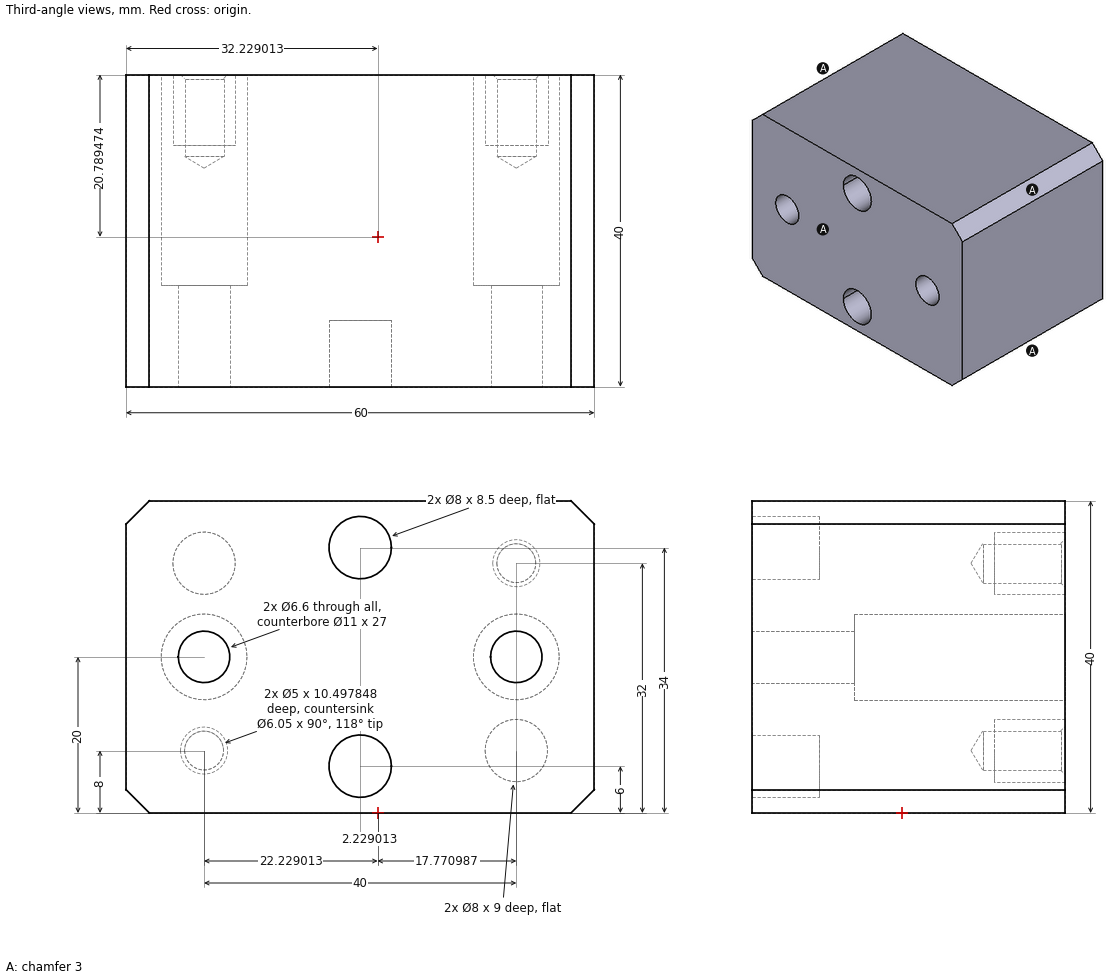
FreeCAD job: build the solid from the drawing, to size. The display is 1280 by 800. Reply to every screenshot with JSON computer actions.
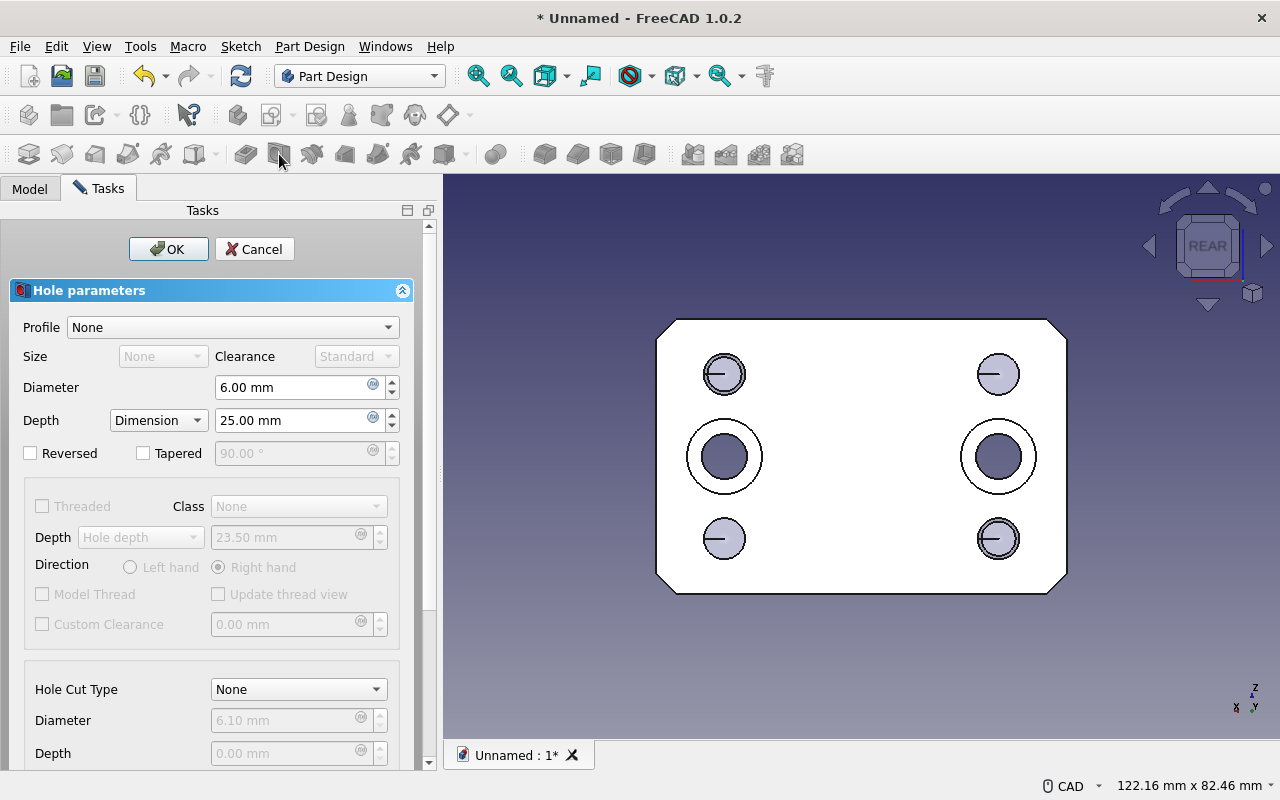
{"action": "triple_click", "coordinate": [300, 388]}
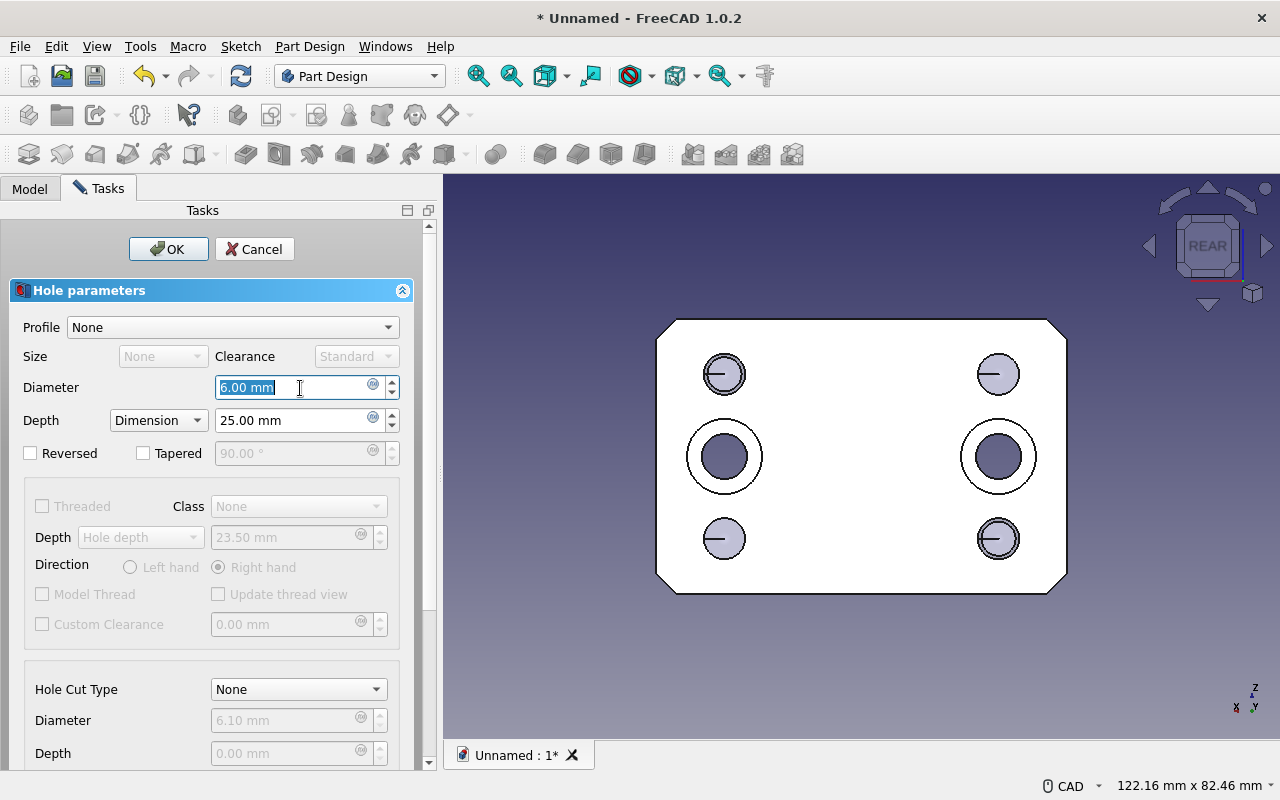
{"action": "type", "text": "8"}
{"action": "key", "text": "Tab"}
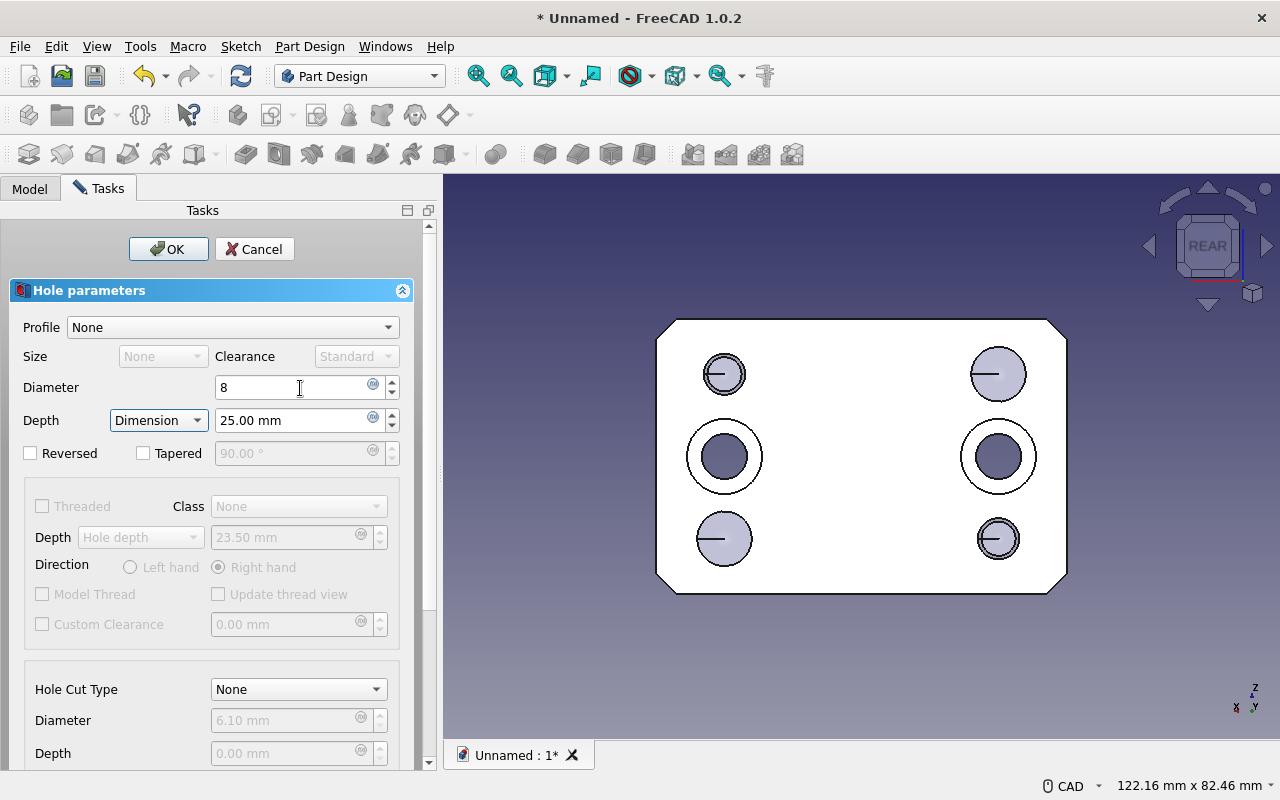
{"action": "triple_click", "coordinate": [300, 420]}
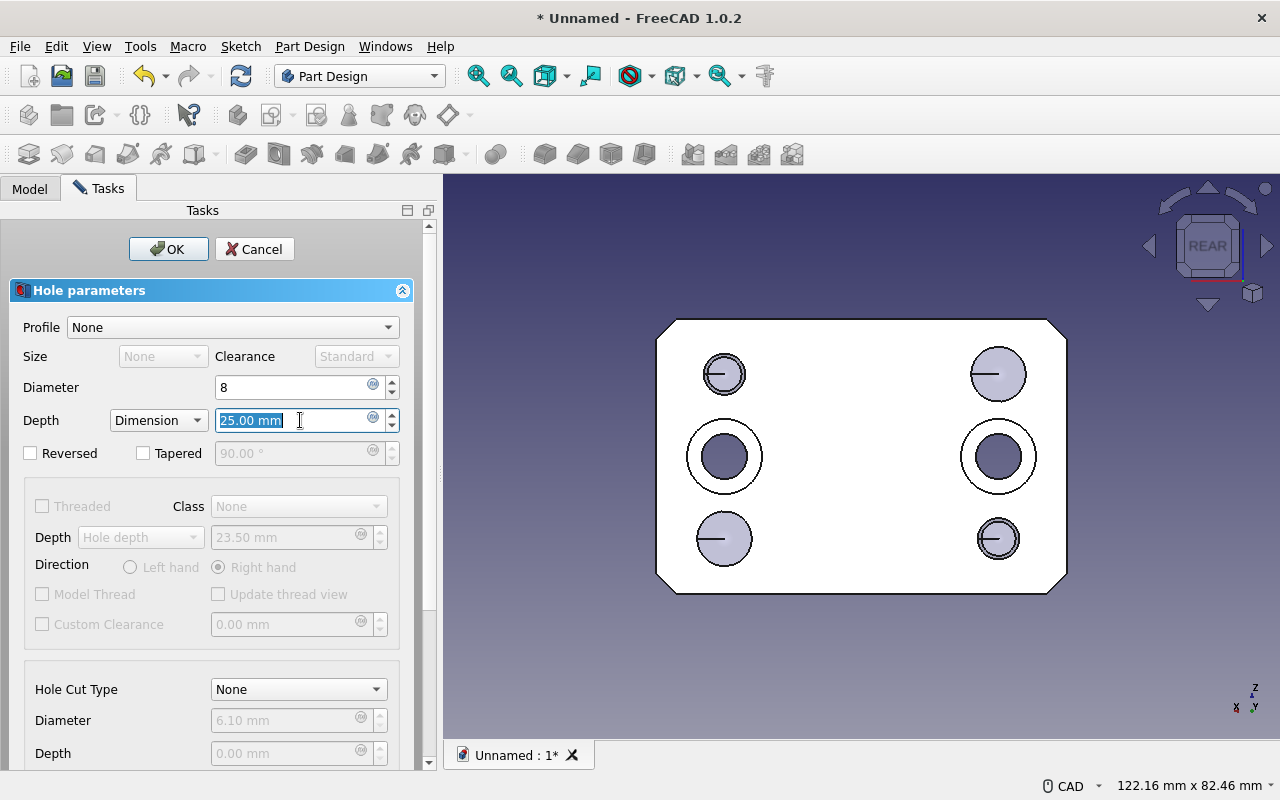
{"action": "type", "text": "9"}
{"action": "key", "text": "Tab"}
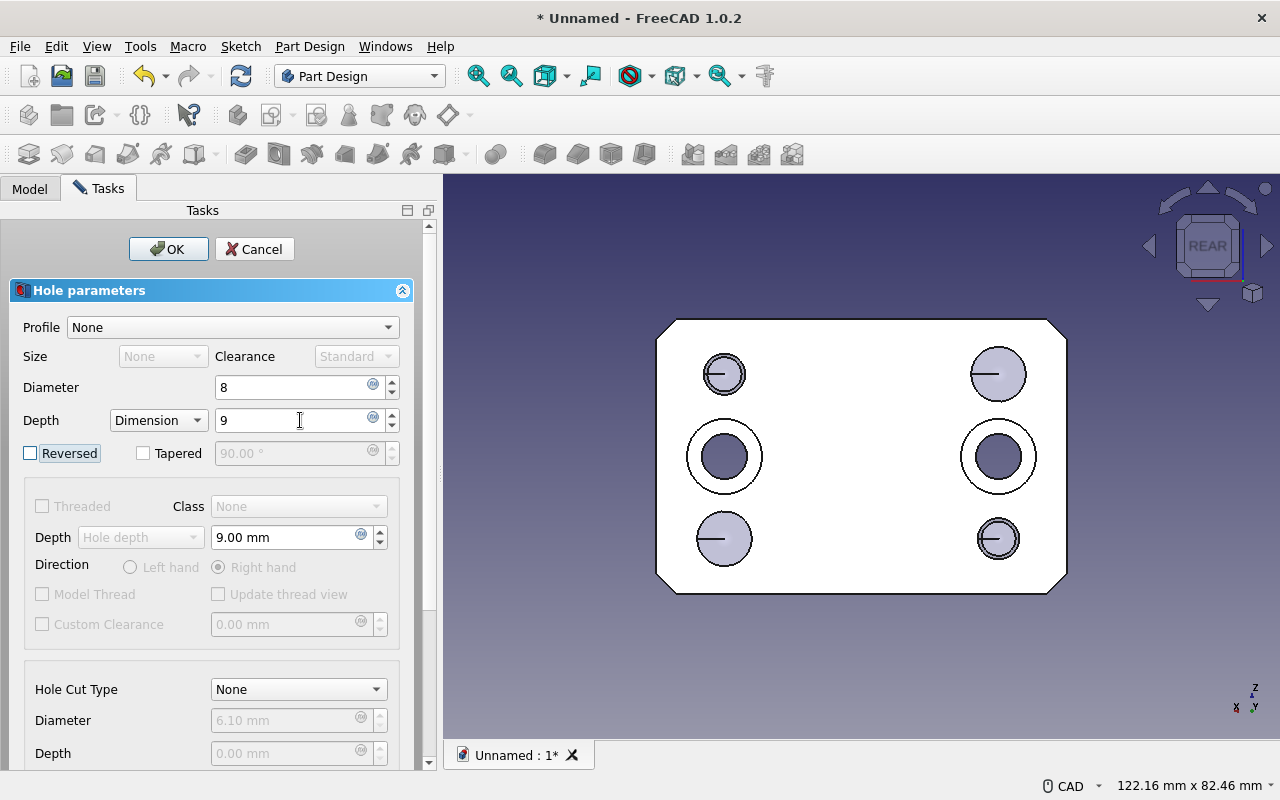
{"action": "scroll", "coordinate": [429, 495], "scroll_direction": "down", "scroll_amount": 3}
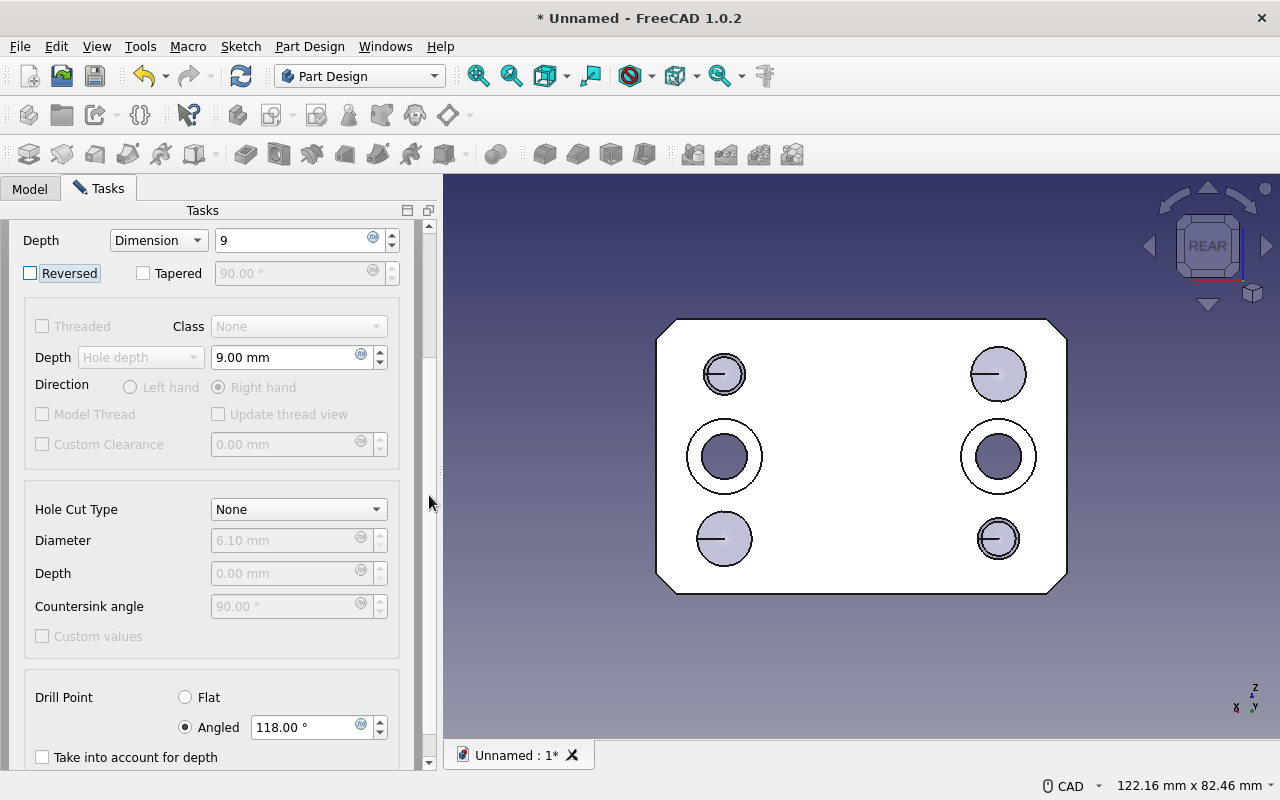
{"action": "left_click", "coordinate": [186, 695]}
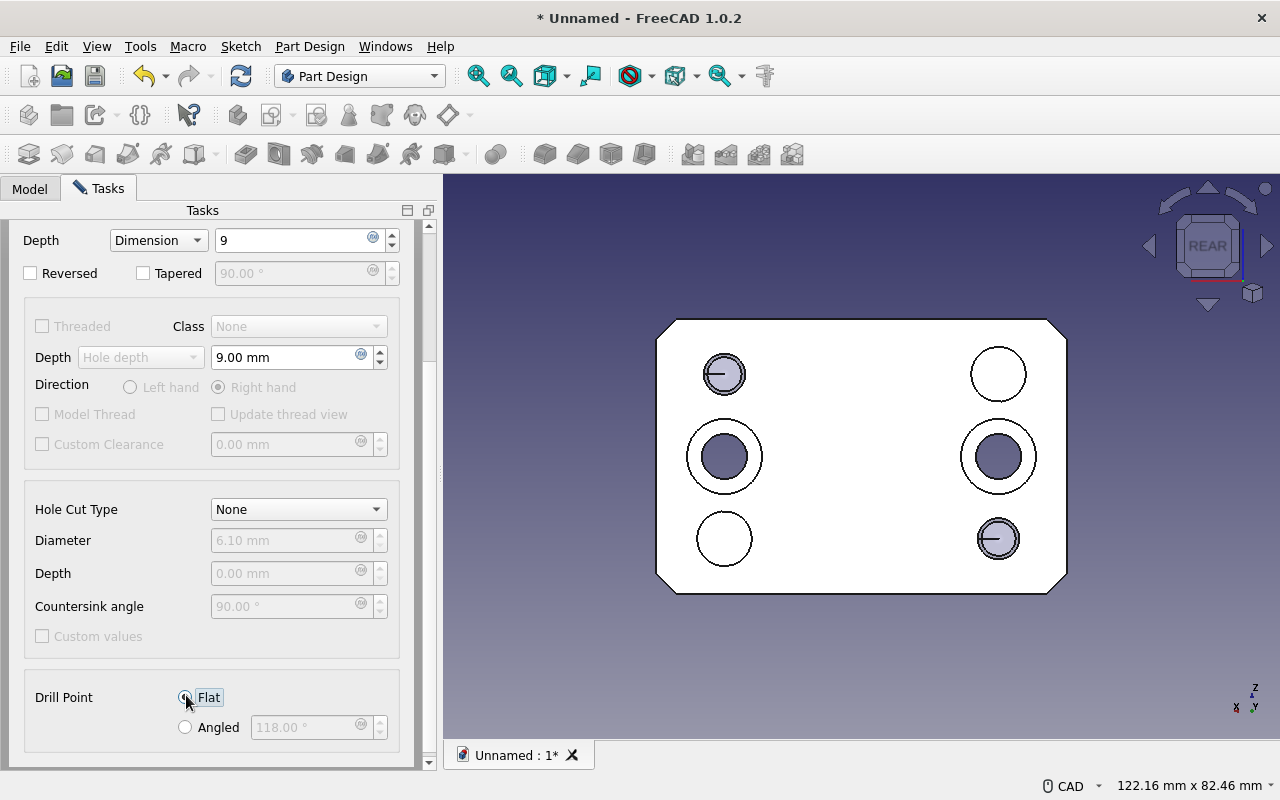
{"action": "scroll", "coordinate": [429, 495], "scroll_direction": "up", "scroll_amount": 4}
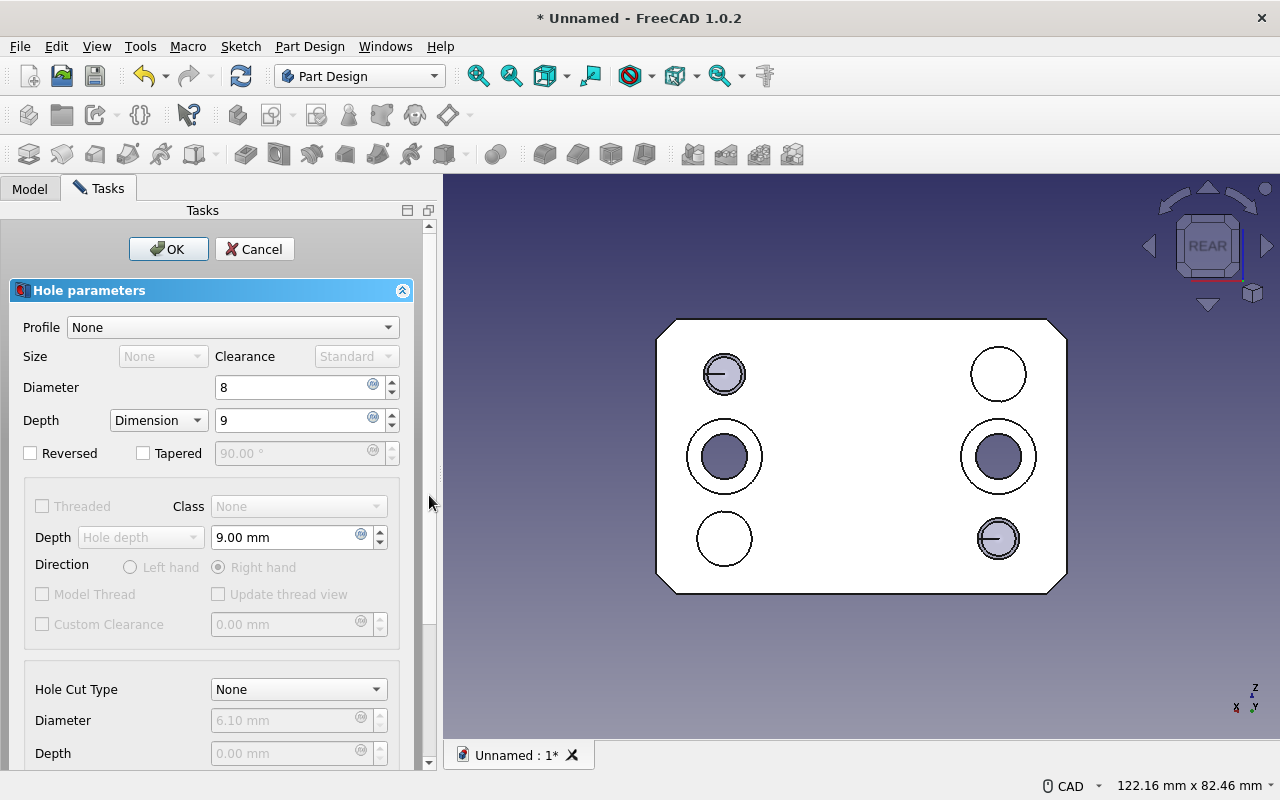
{"action": "left_click", "coordinate": [169, 249]}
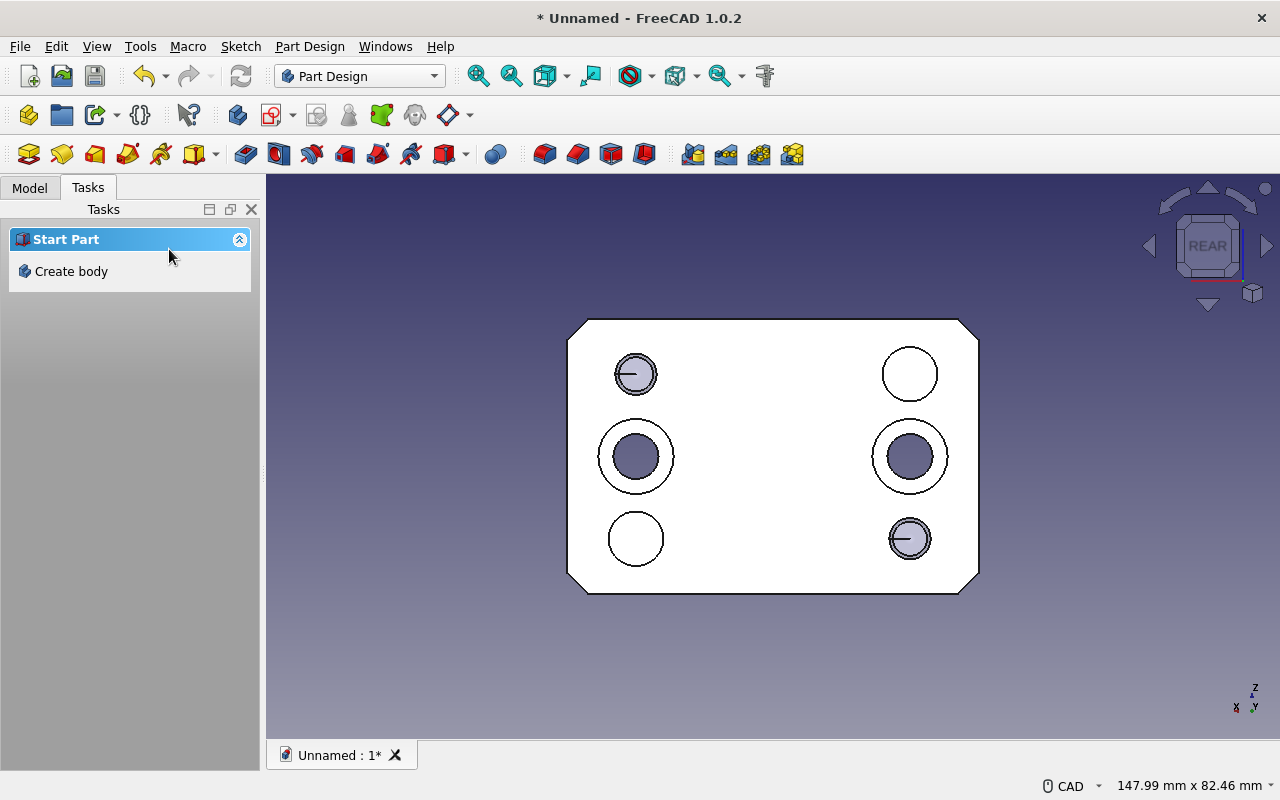
{"action": "key", "text": "0"}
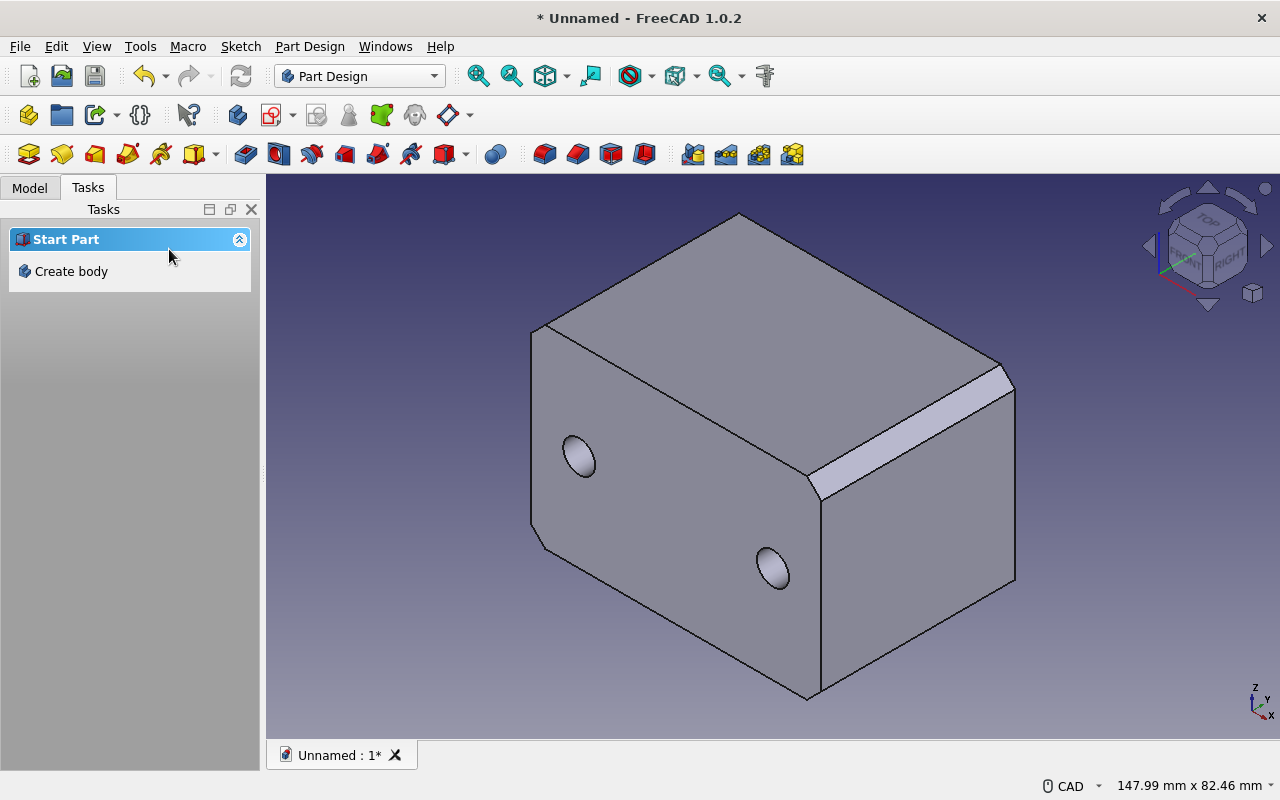
{"action": "left_click", "coordinate": [676, 511]}